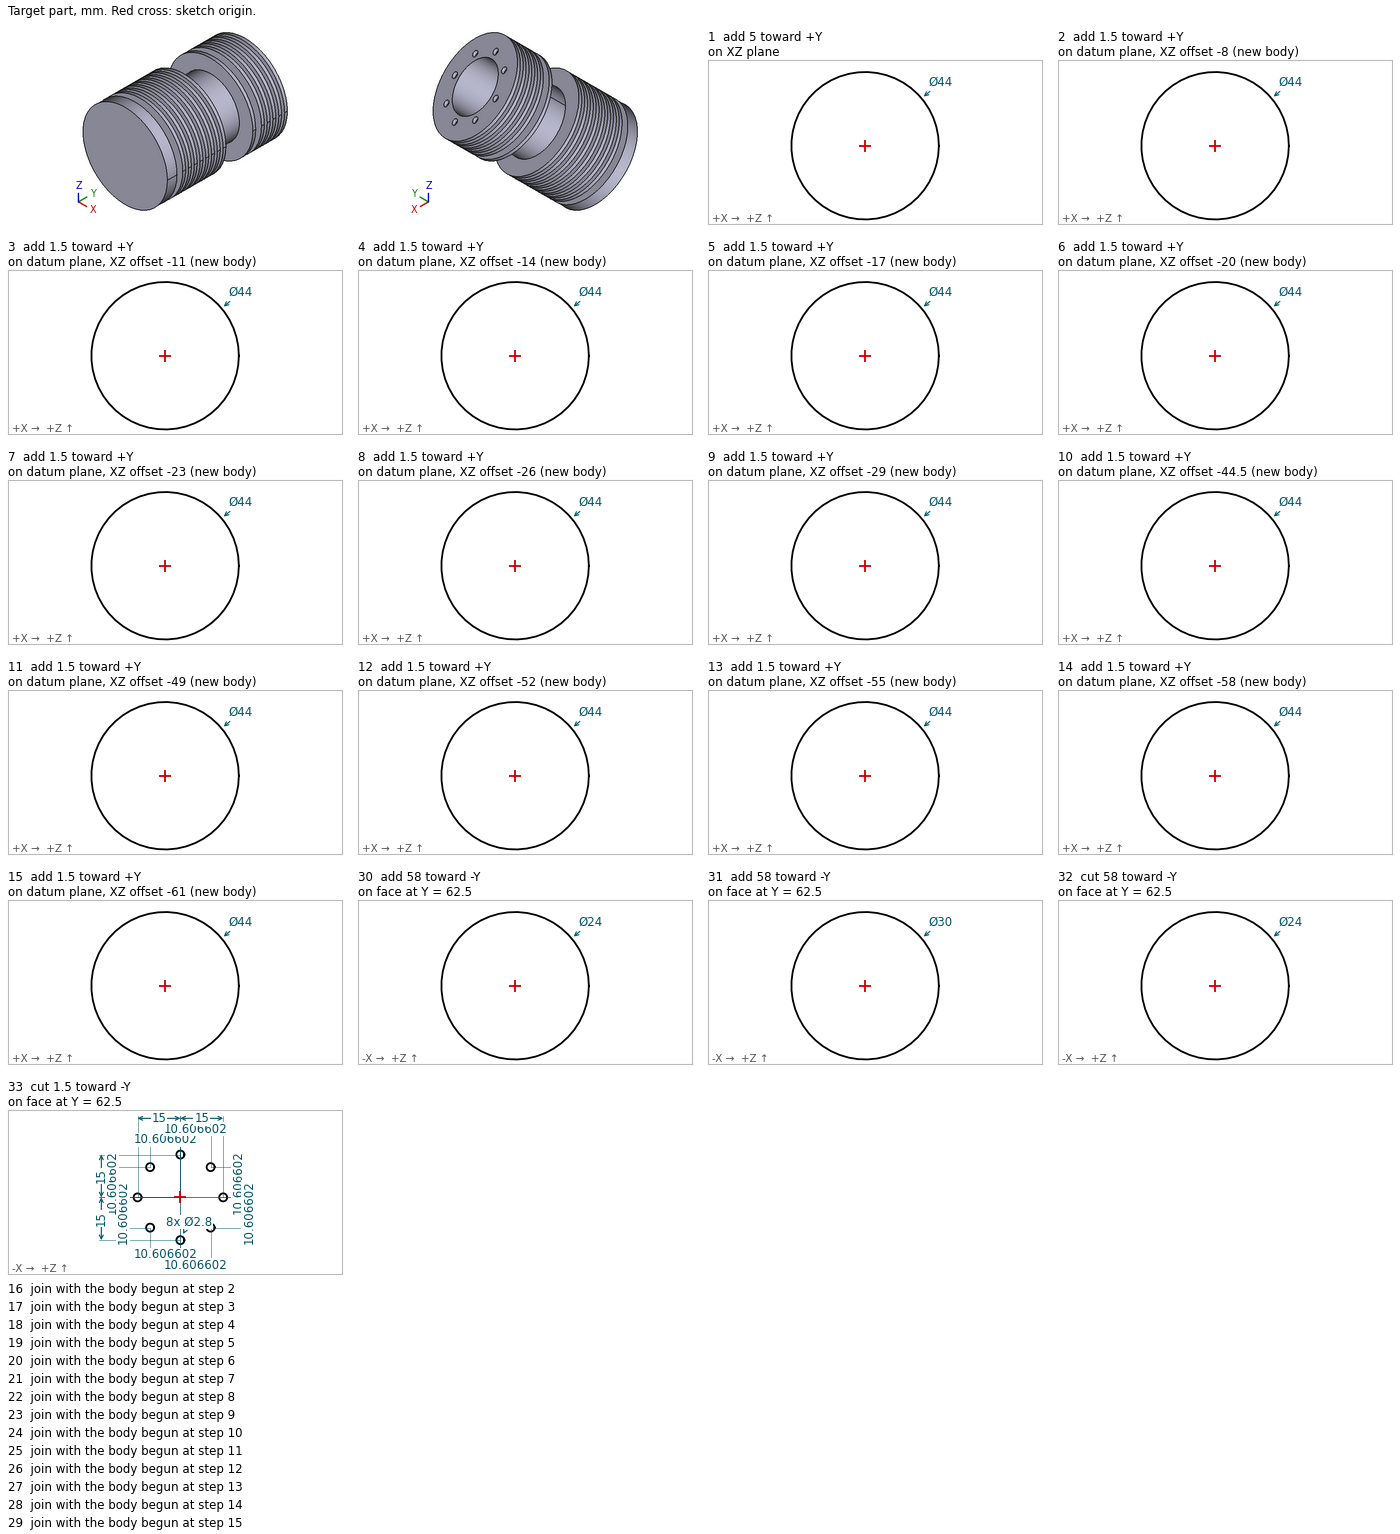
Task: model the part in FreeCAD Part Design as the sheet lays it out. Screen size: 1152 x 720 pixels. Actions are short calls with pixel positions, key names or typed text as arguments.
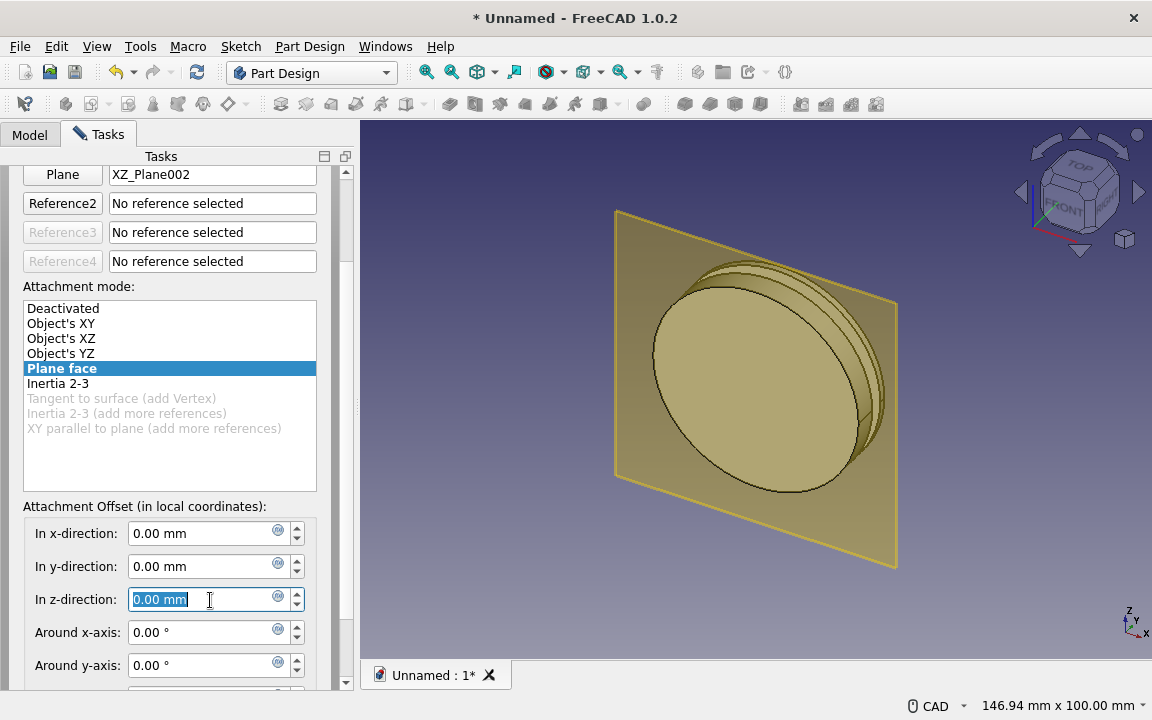
text(-11)
key(Tab)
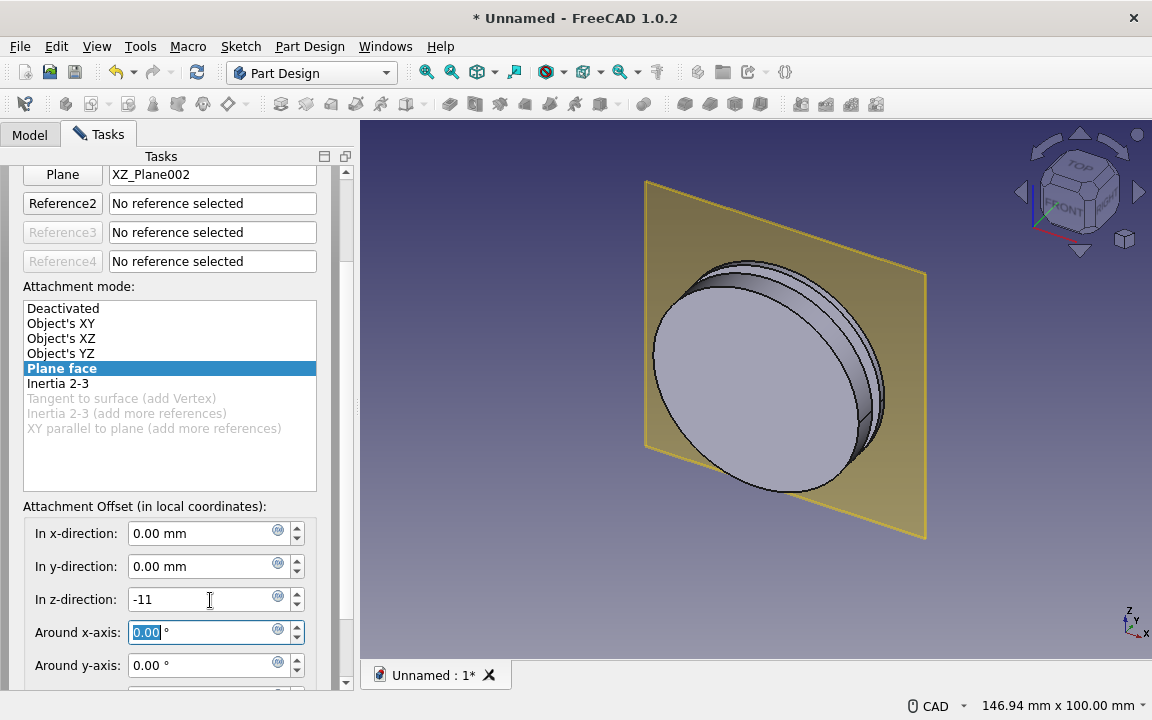
scroll(346, 428, up, 3)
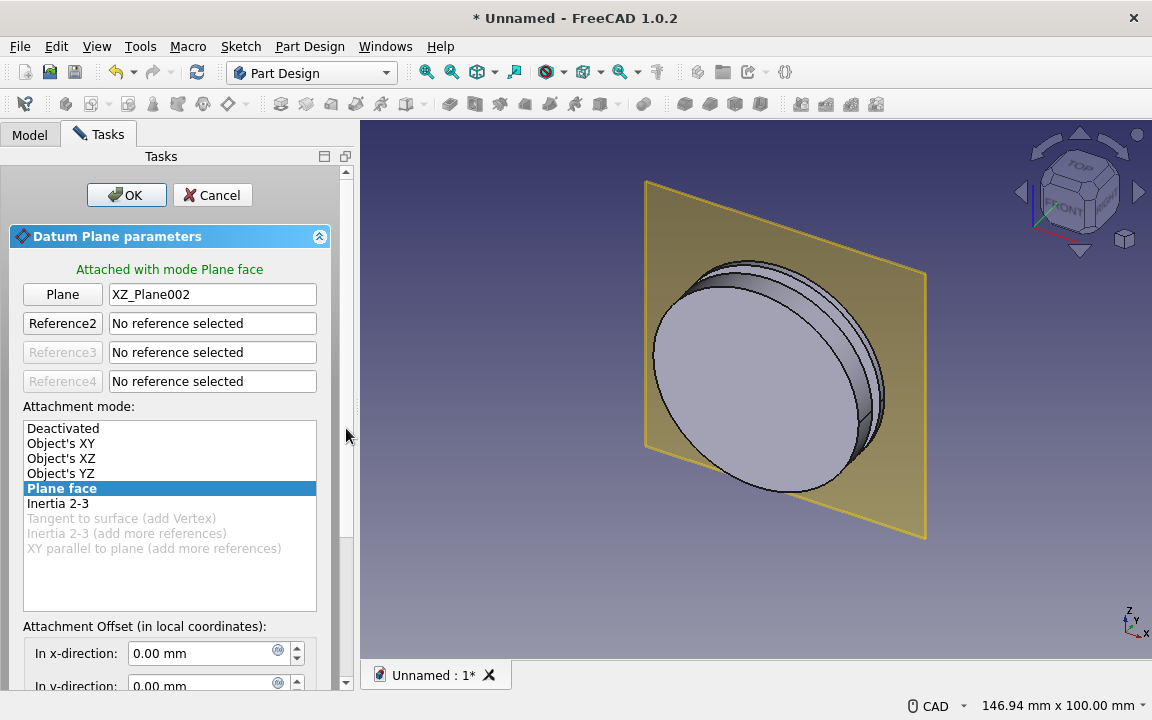
click(127, 195)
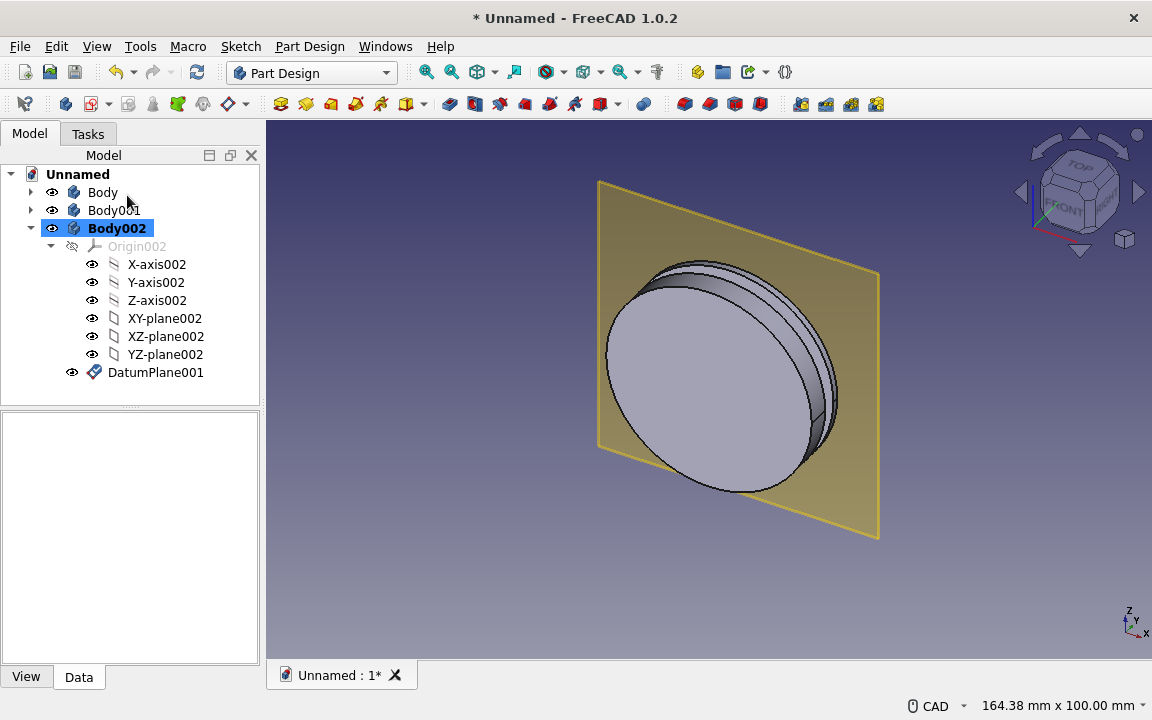
click(117, 372)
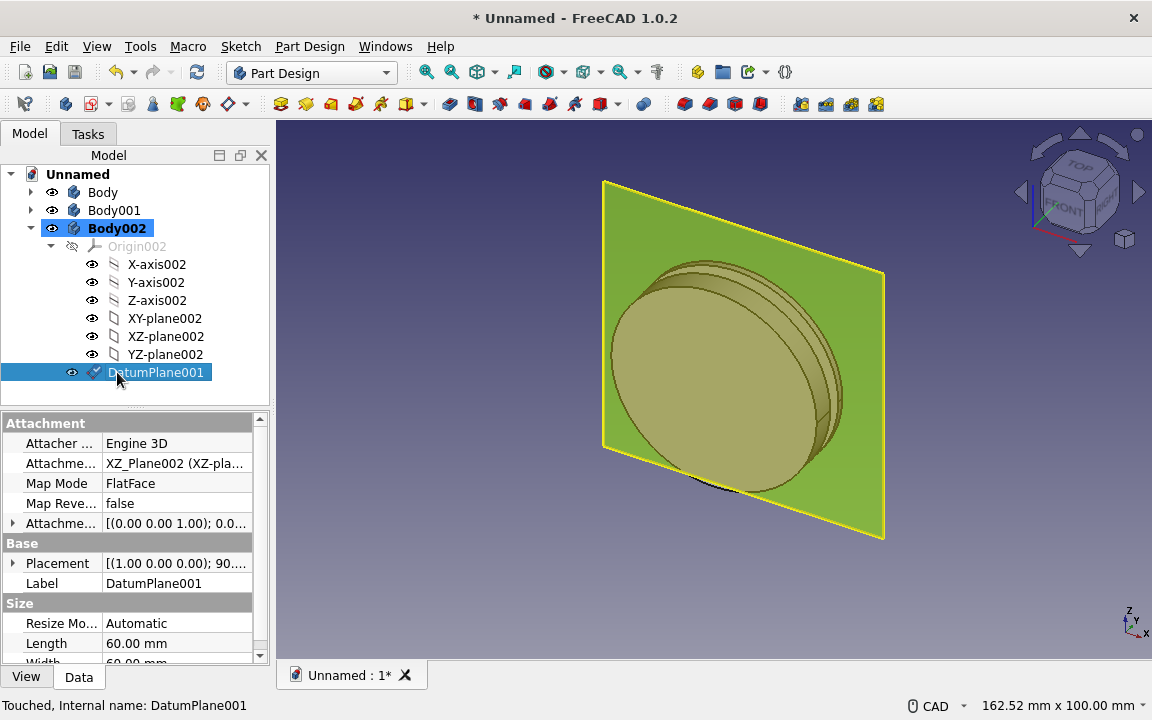
click(90, 104)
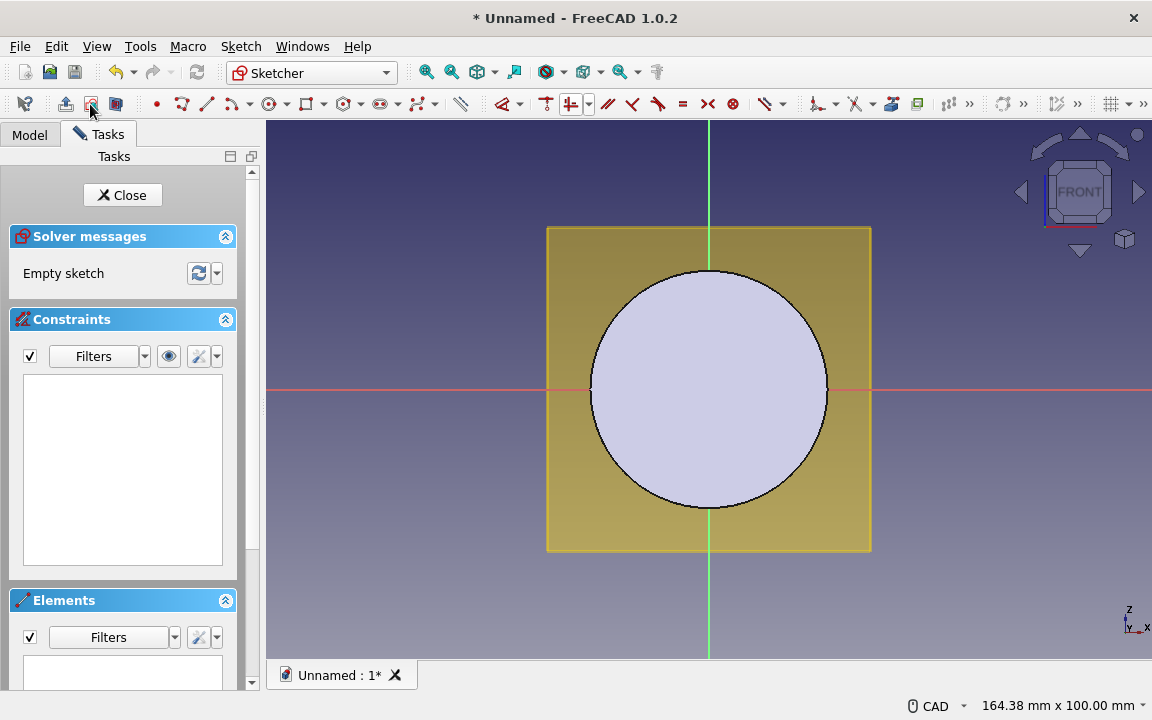
scroll(848, 390, up, 2)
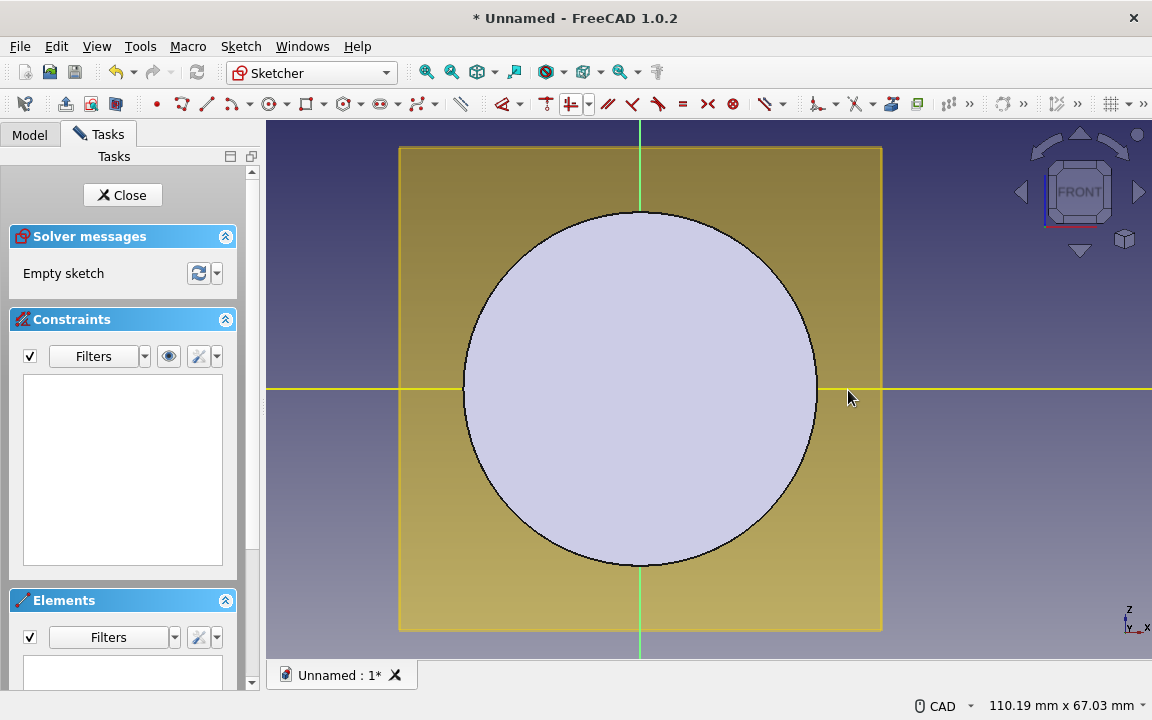
key(g)
key(c)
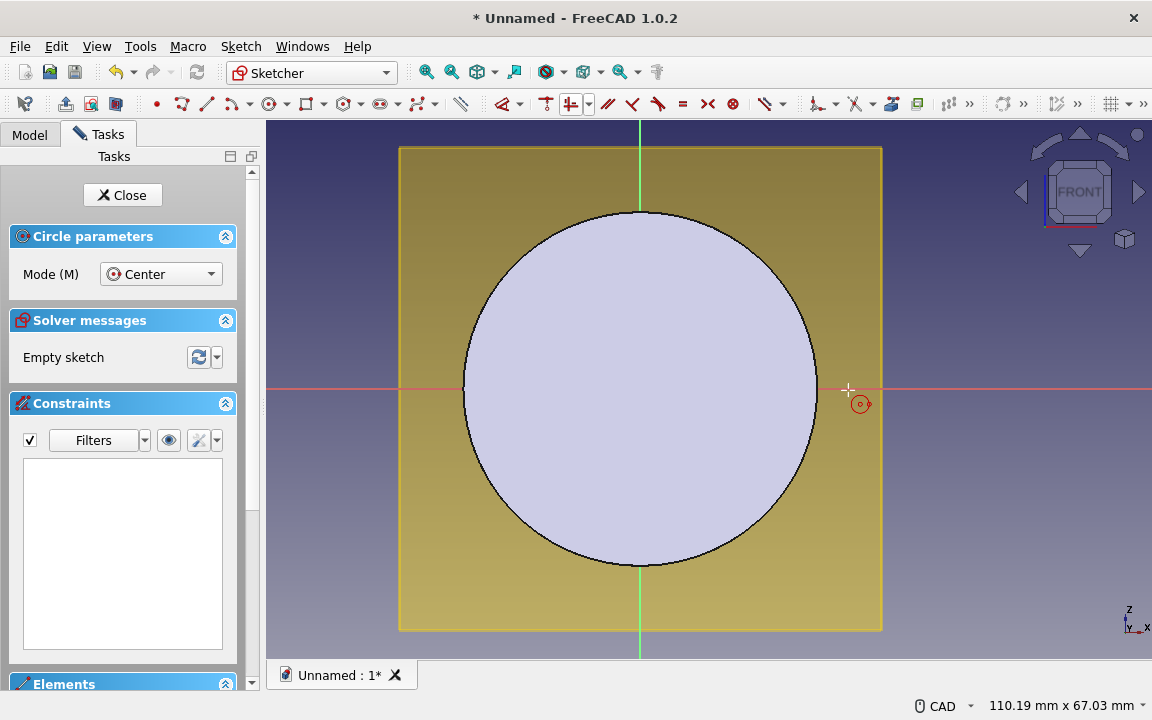
click(640, 389)
click(765, 264)
key(Escape)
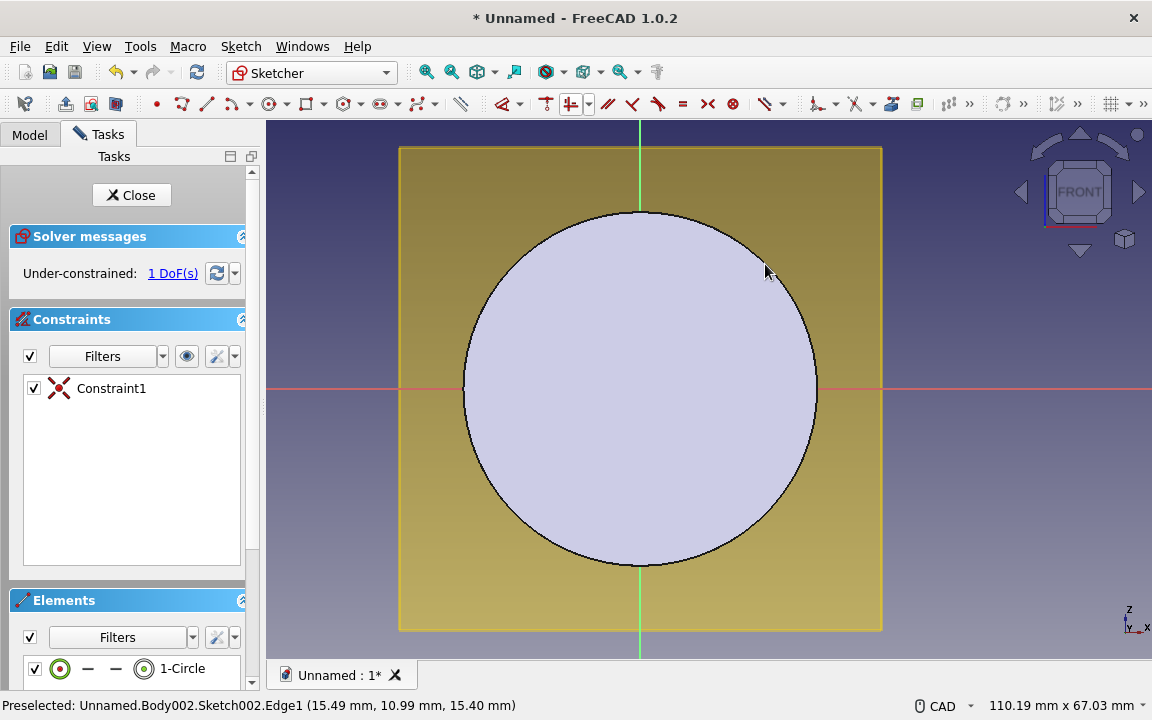
click(764, 264)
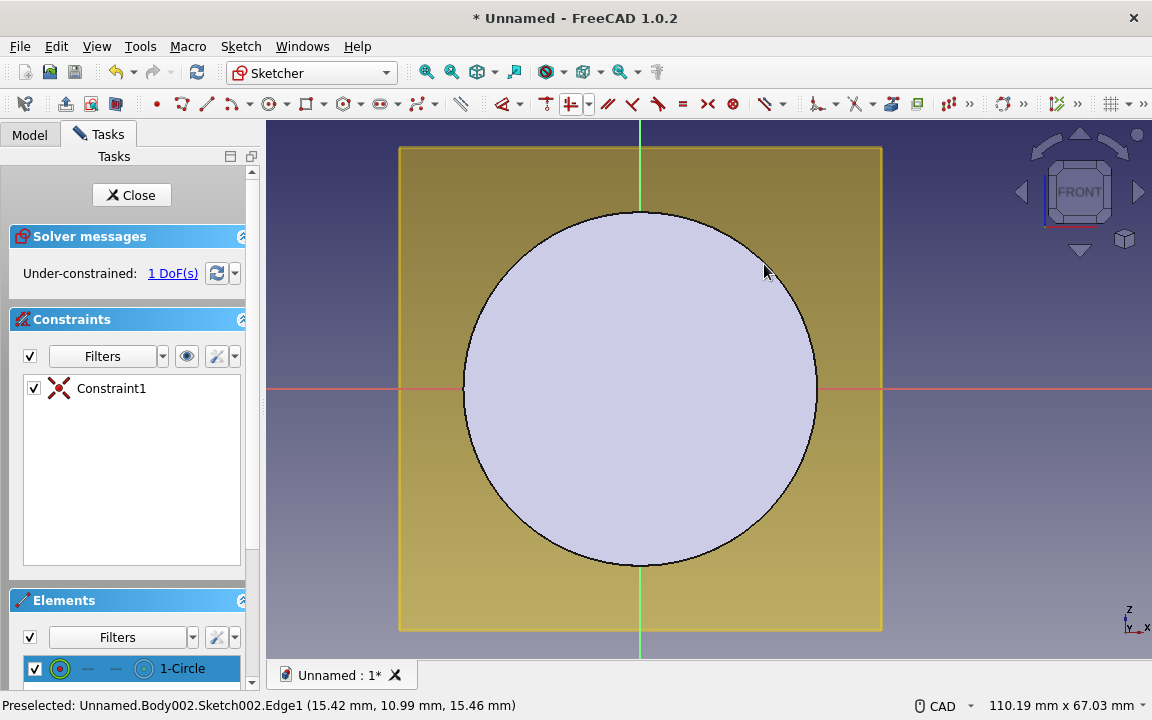
click(520, 104)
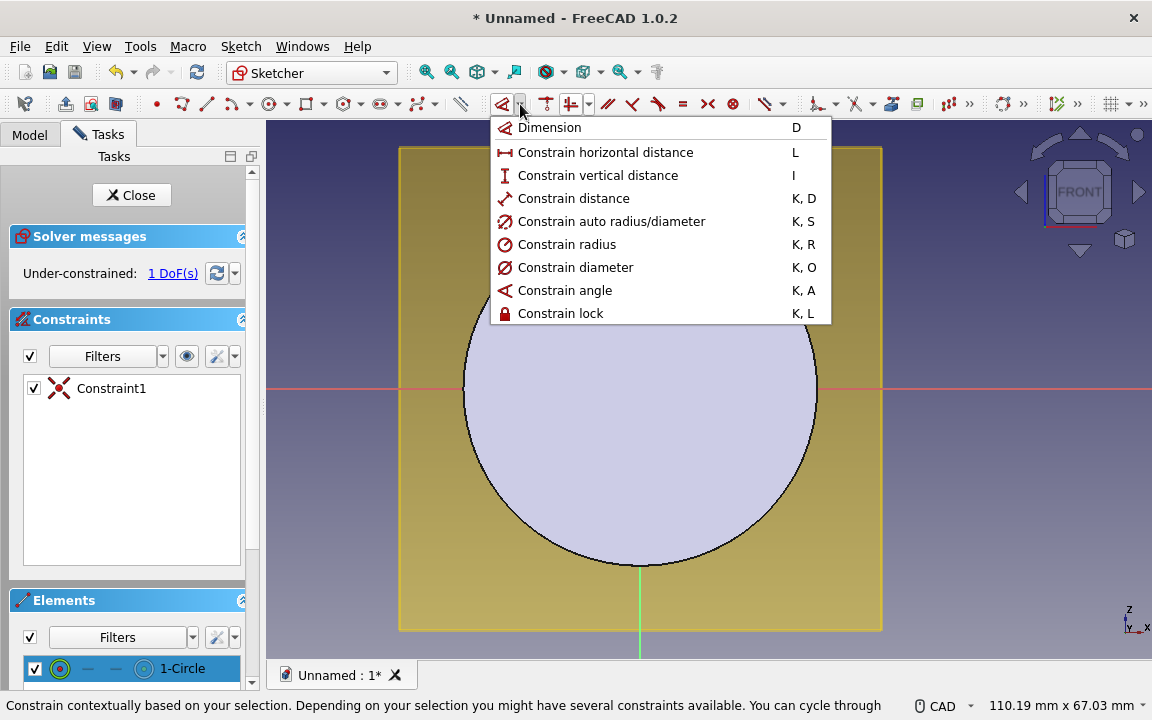
click(661, 268)